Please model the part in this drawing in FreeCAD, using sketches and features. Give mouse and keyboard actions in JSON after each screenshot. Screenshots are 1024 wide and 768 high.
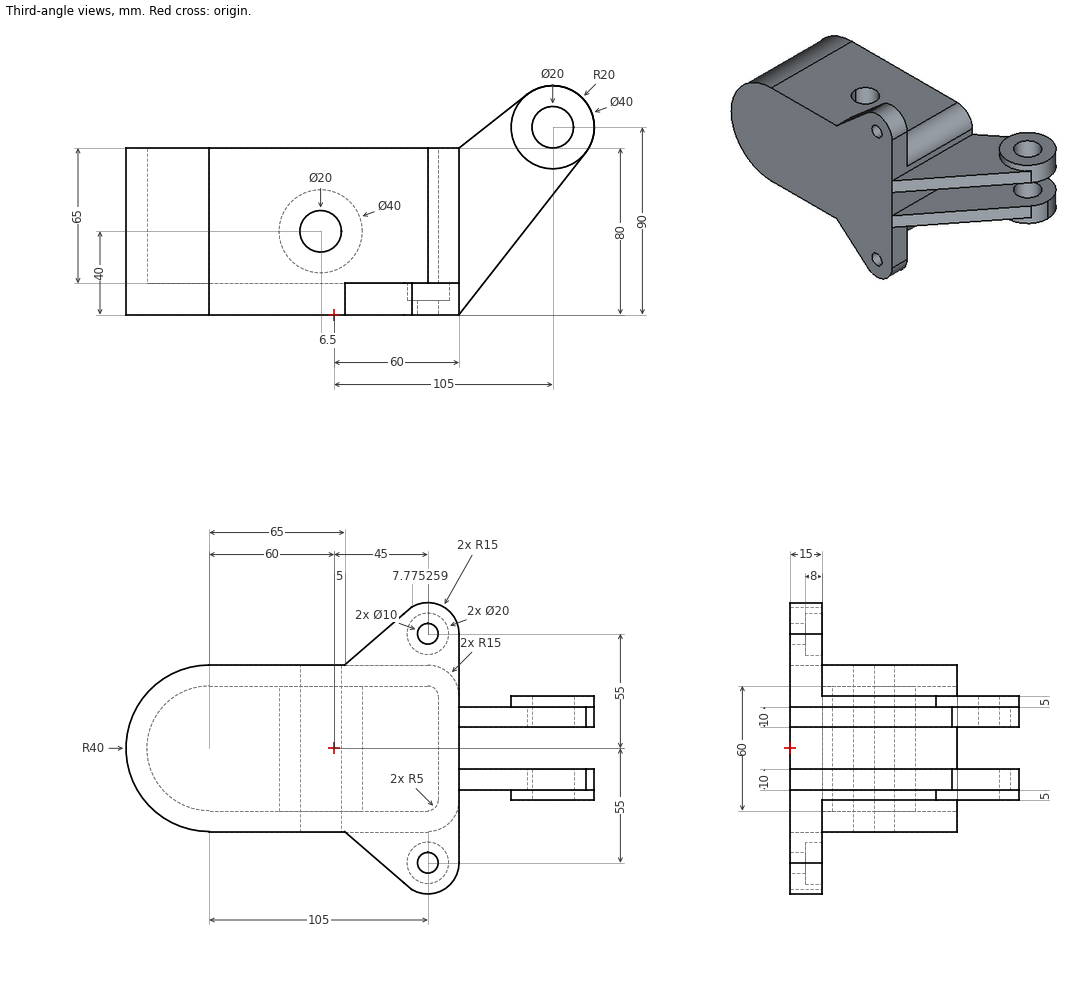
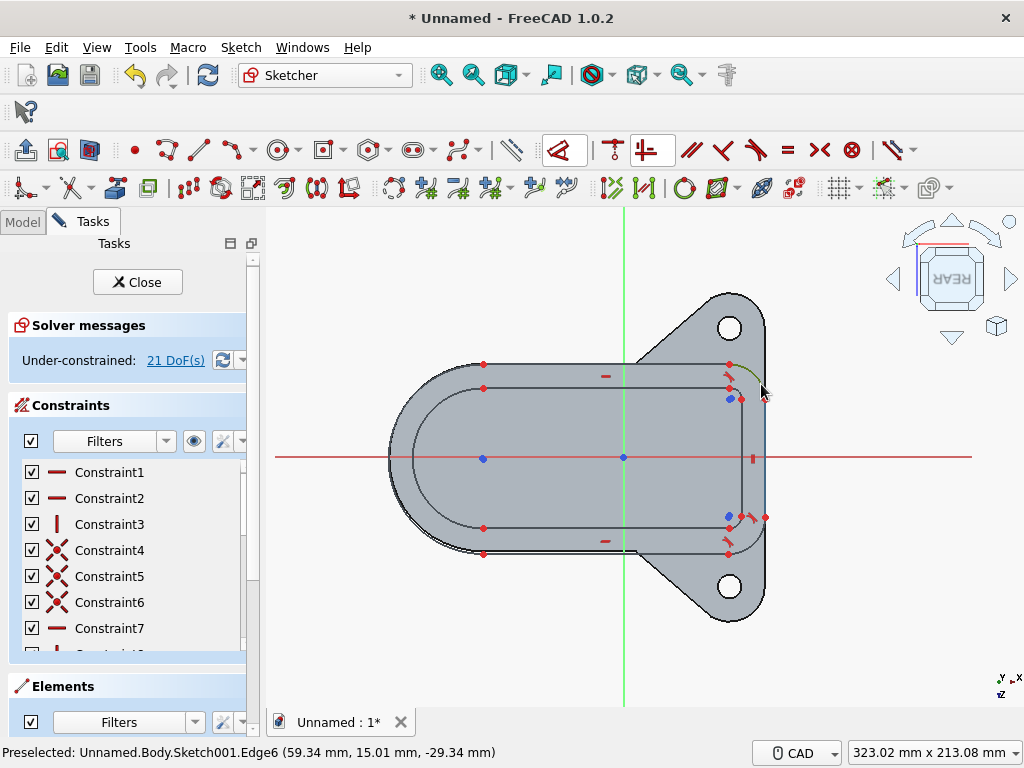
{"action": "left_click", "coordinate": [756, 150]}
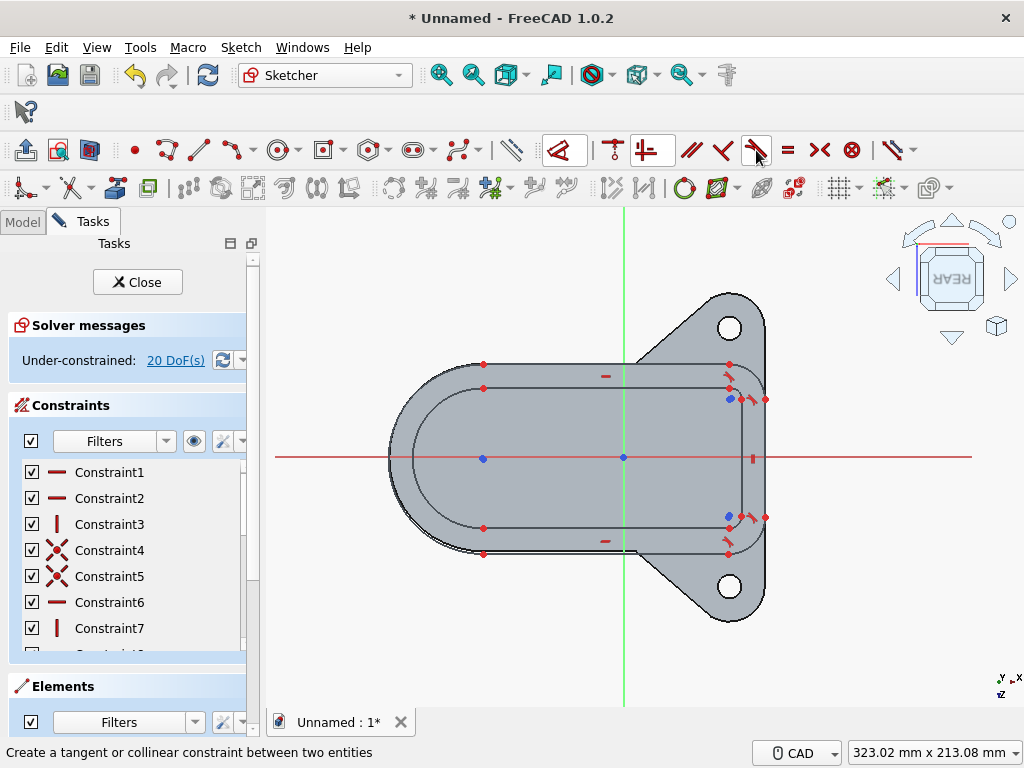
{"action": "left_click", "coordinate": [557, 388]}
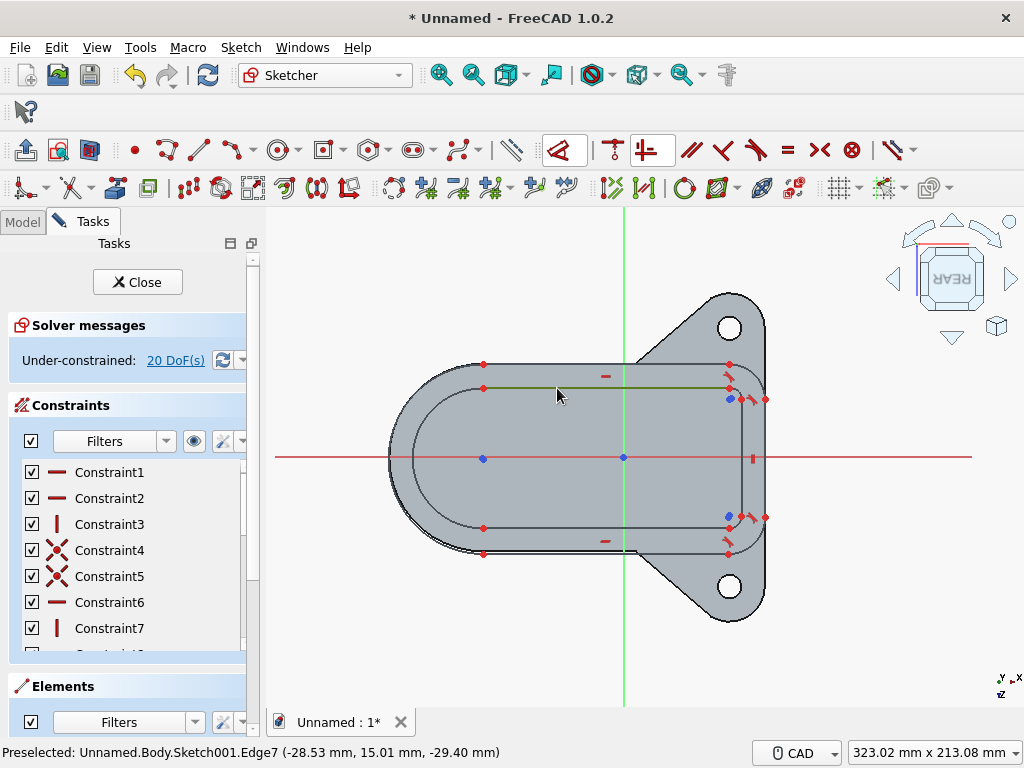
{"action": "scroll", "coordinate": [738, 391], "scroll_direction": "up", "scroll_amount": 3}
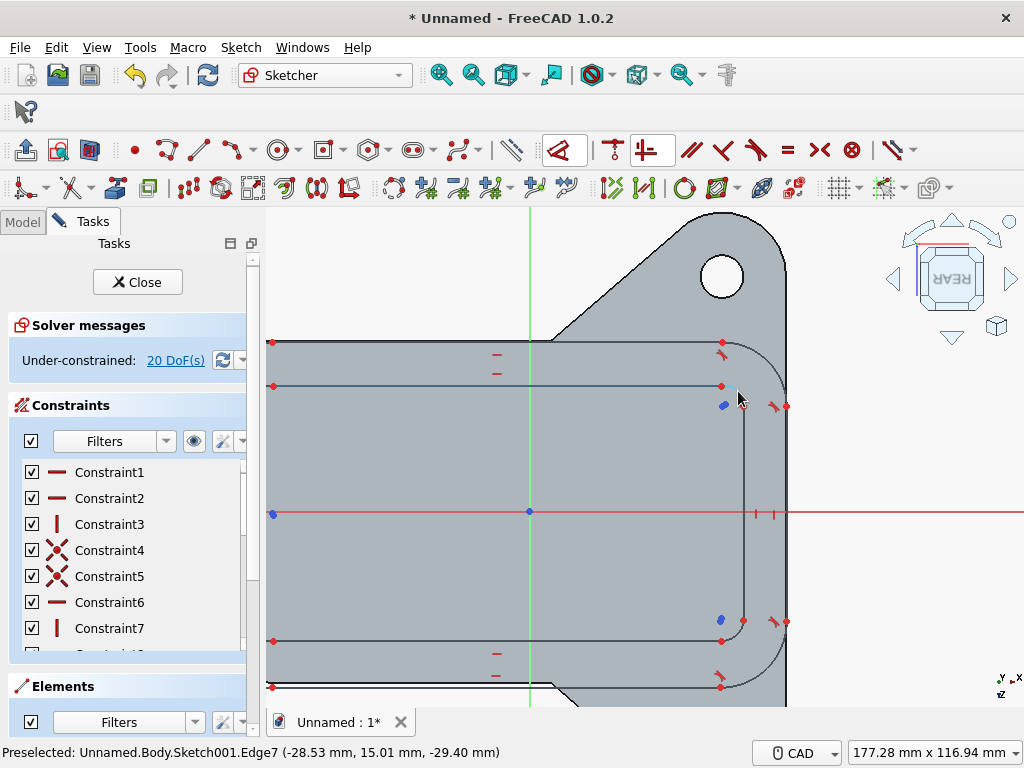
{"action": "left_click", "coordinate": [738, 391]}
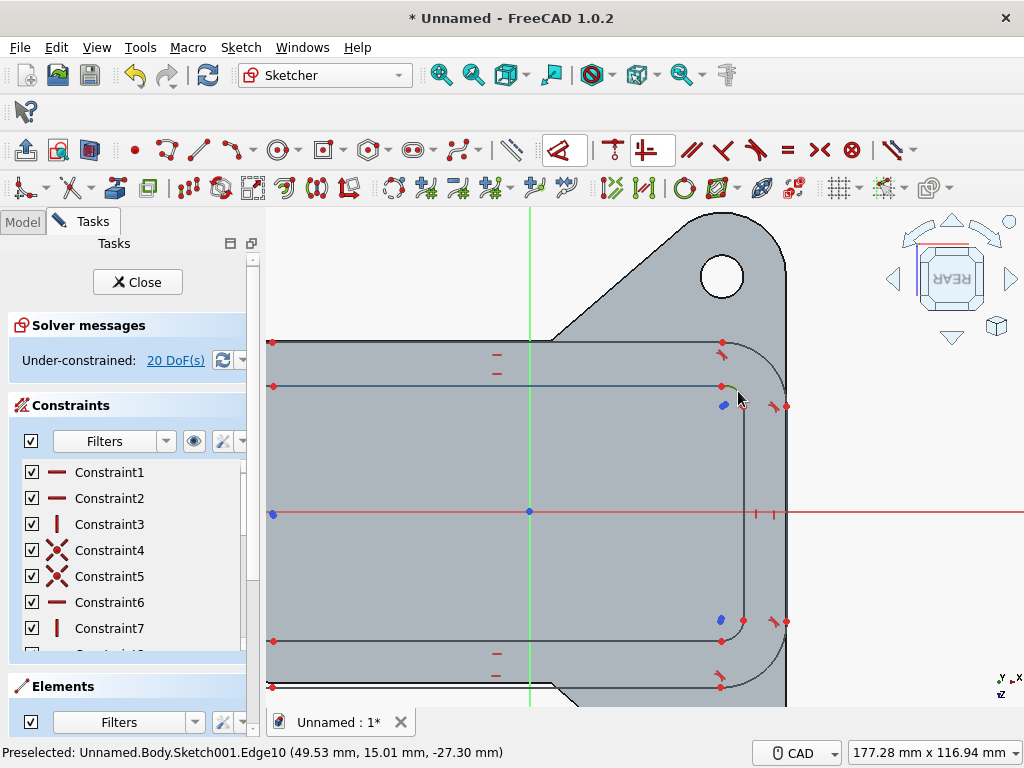
{"action": "left_click", "coordinate": [756, 150]}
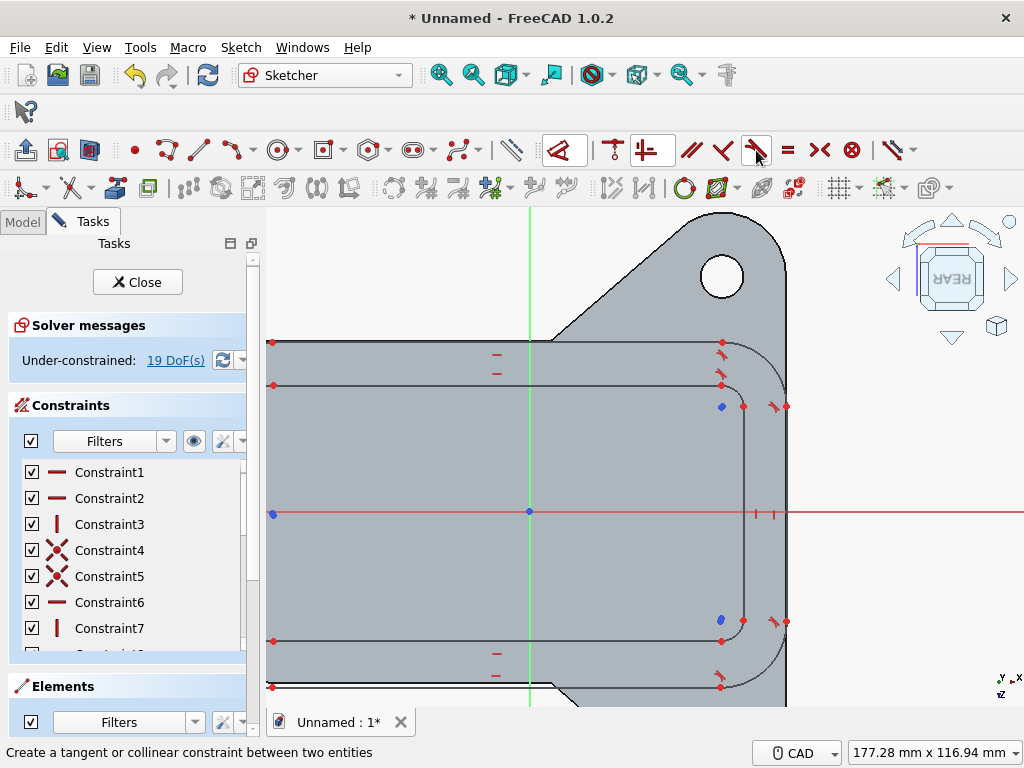
{"action": "left_click", "coordinate": [408, 386]}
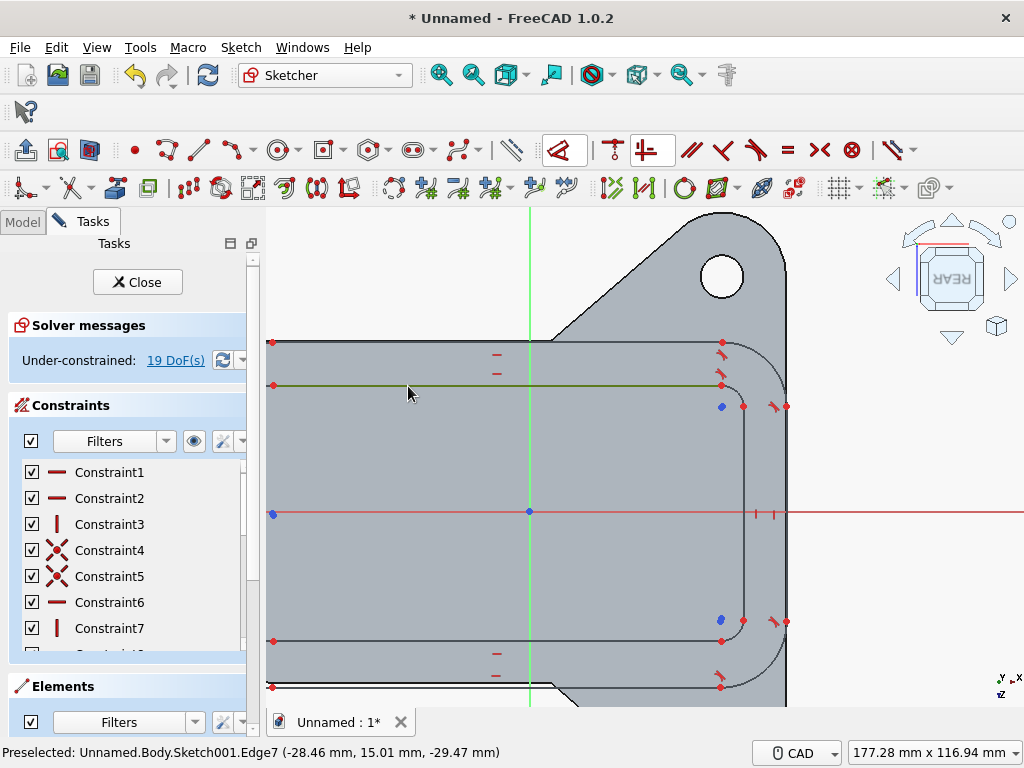
{"action": "scroll", "coordinate": [737, 390], "scroll_direction": "down", "scroll_amount": 3}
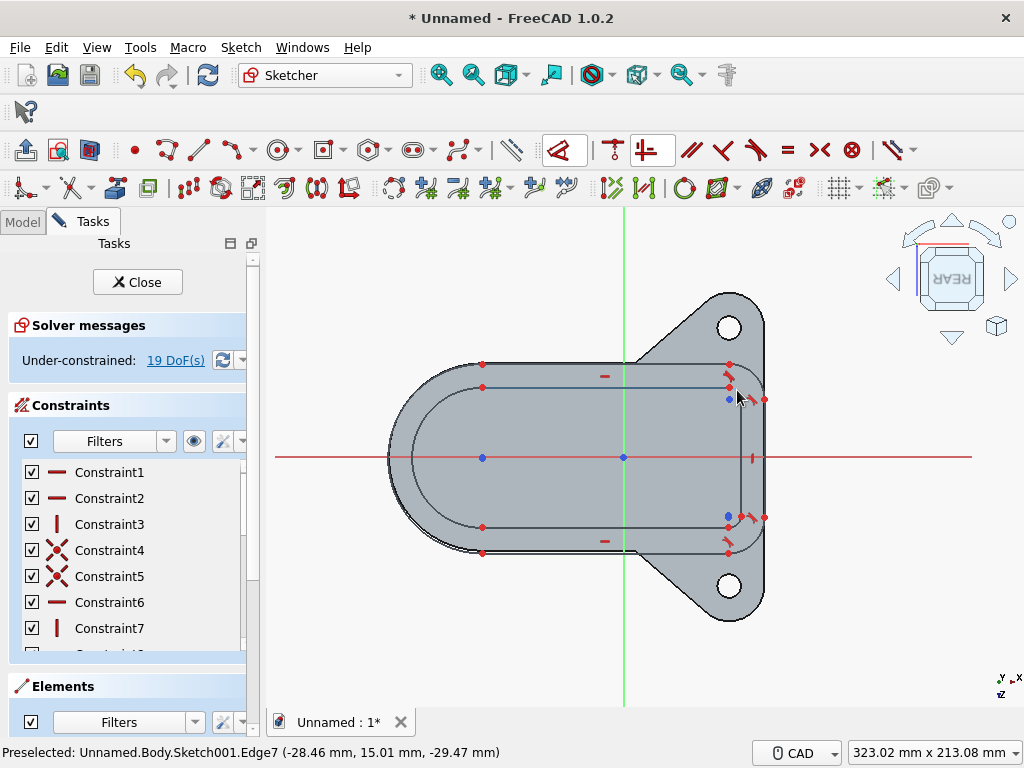
{"action": "left_click", "coordinate": [426, 417]}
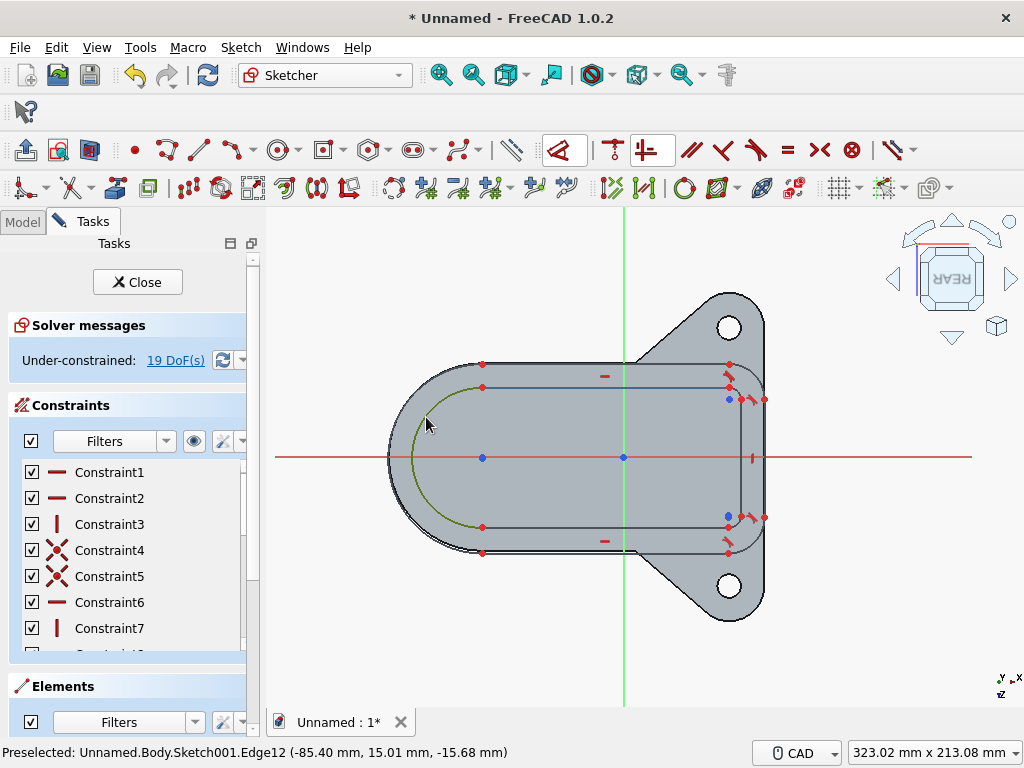
{"action": "left_click", "coordinate": [756, 150]}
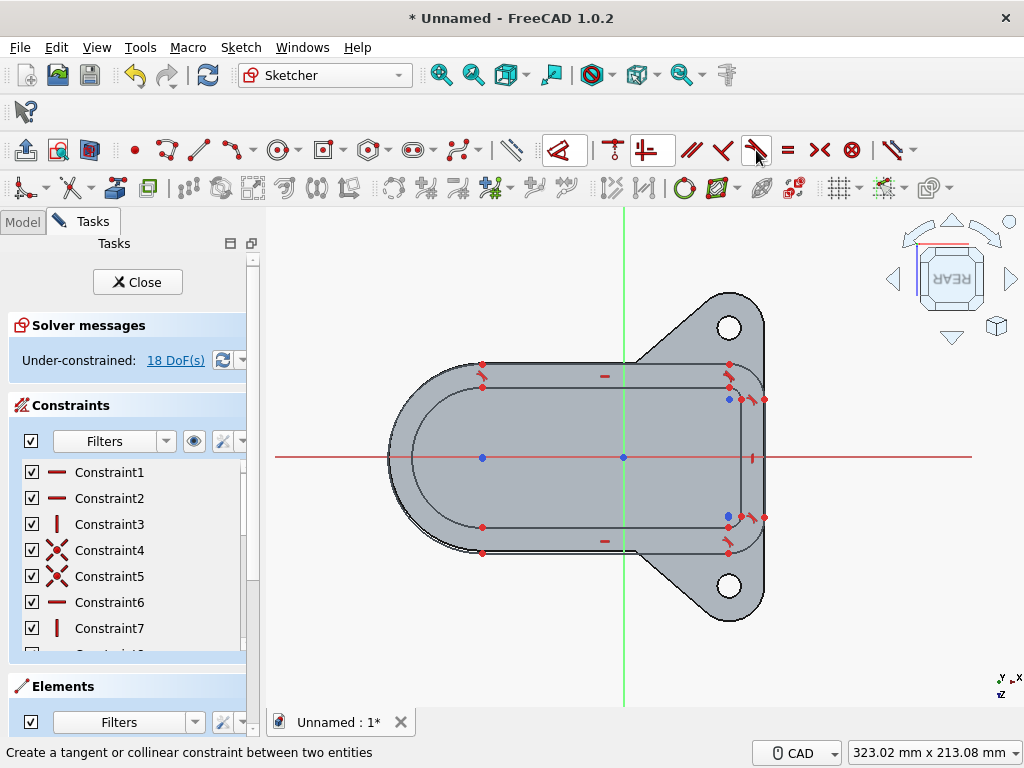
{"action": "left_click", "coordinate": [741, 434]}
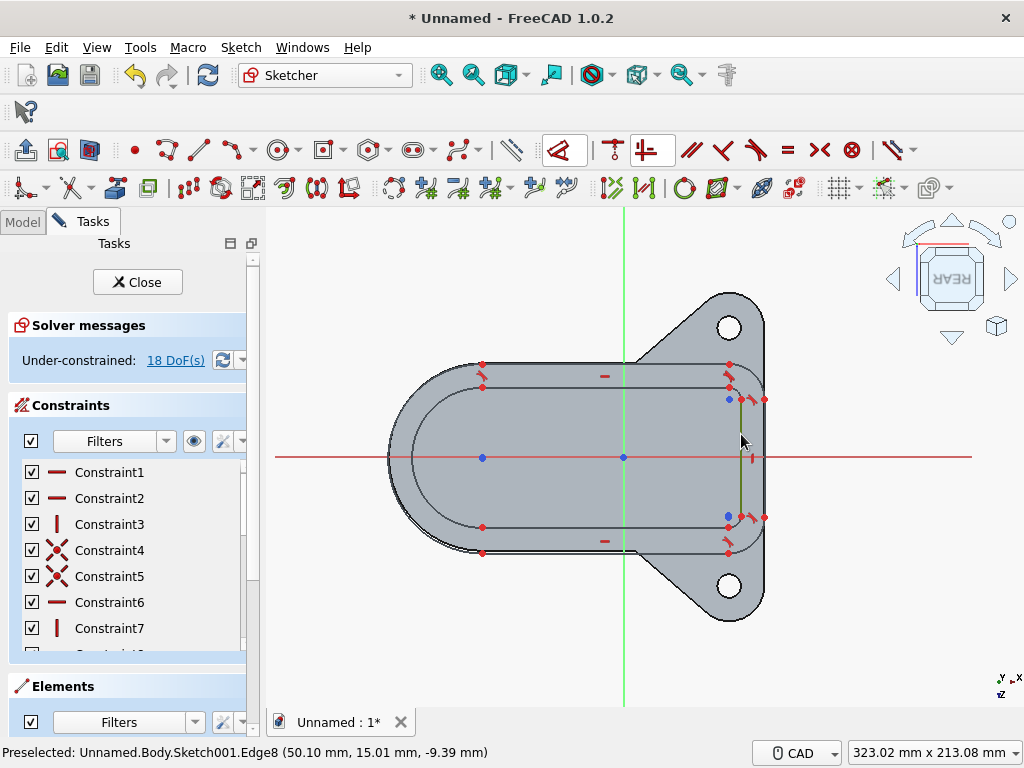
{"action": "scroll", "coordinate": [737, 391], "scroll_direction": "up", "scroll_amount": 3}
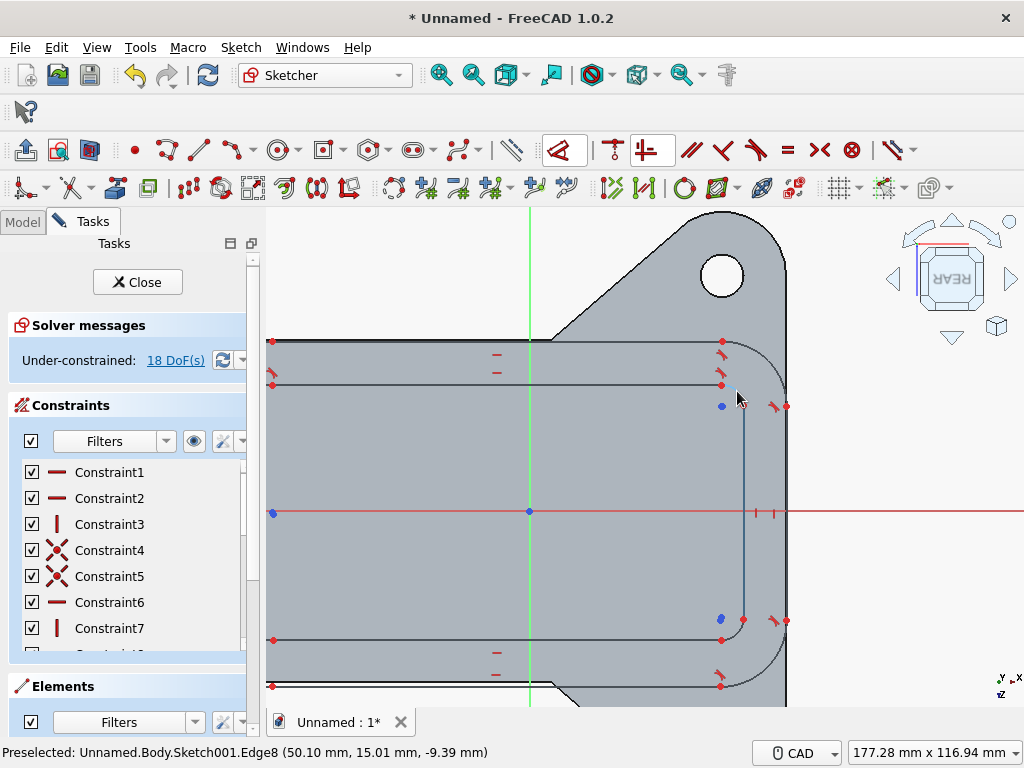
{"action": "left_click", "coordinate": [737, 391]}